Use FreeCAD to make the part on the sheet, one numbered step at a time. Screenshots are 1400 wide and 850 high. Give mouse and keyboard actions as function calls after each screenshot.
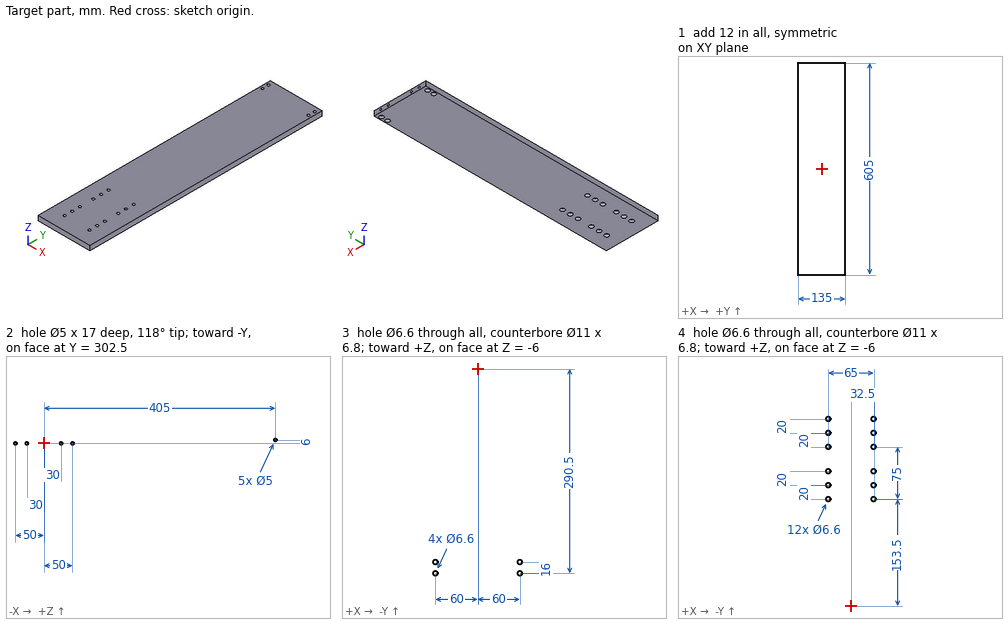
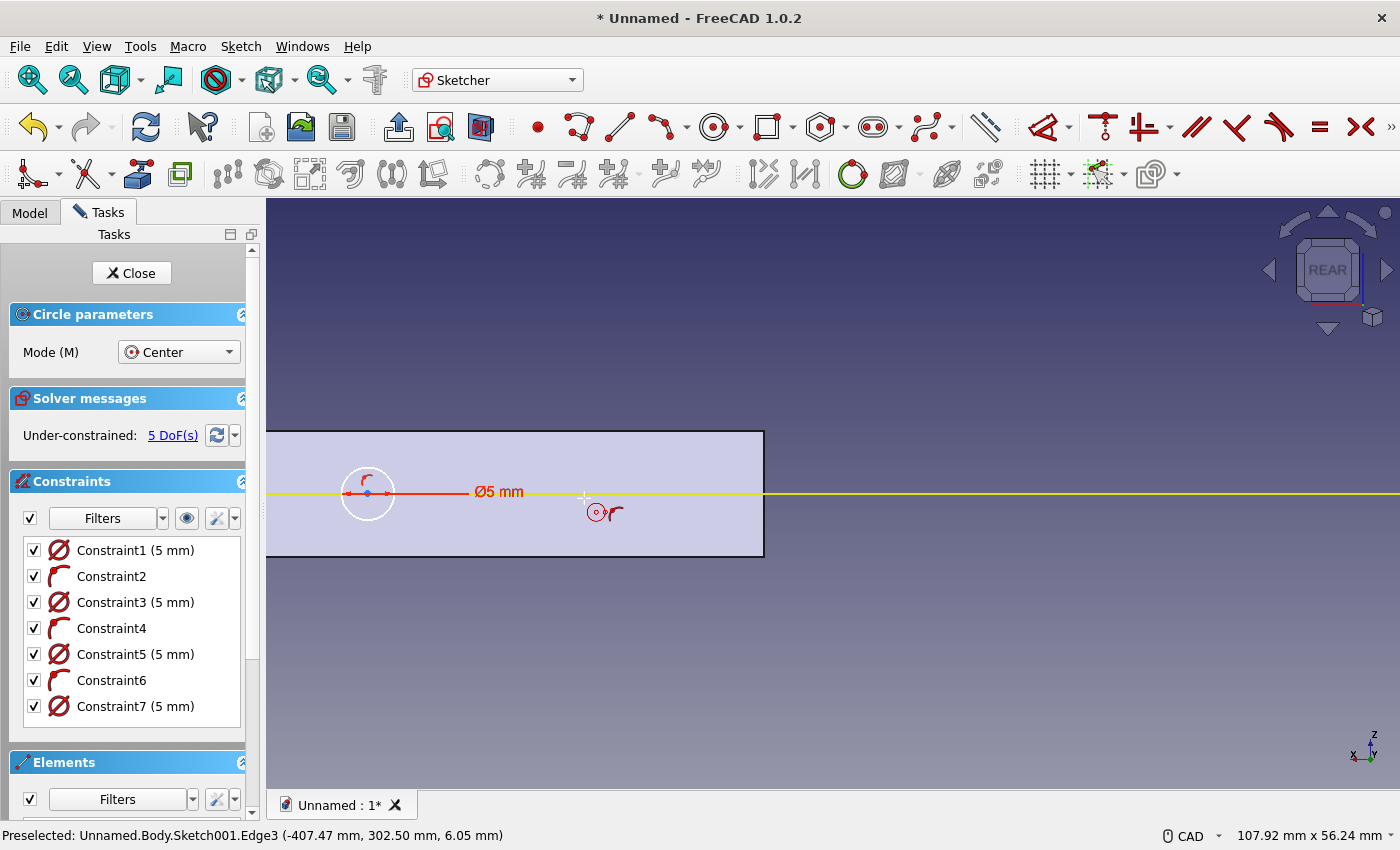
scroll(584, 498, down, 10)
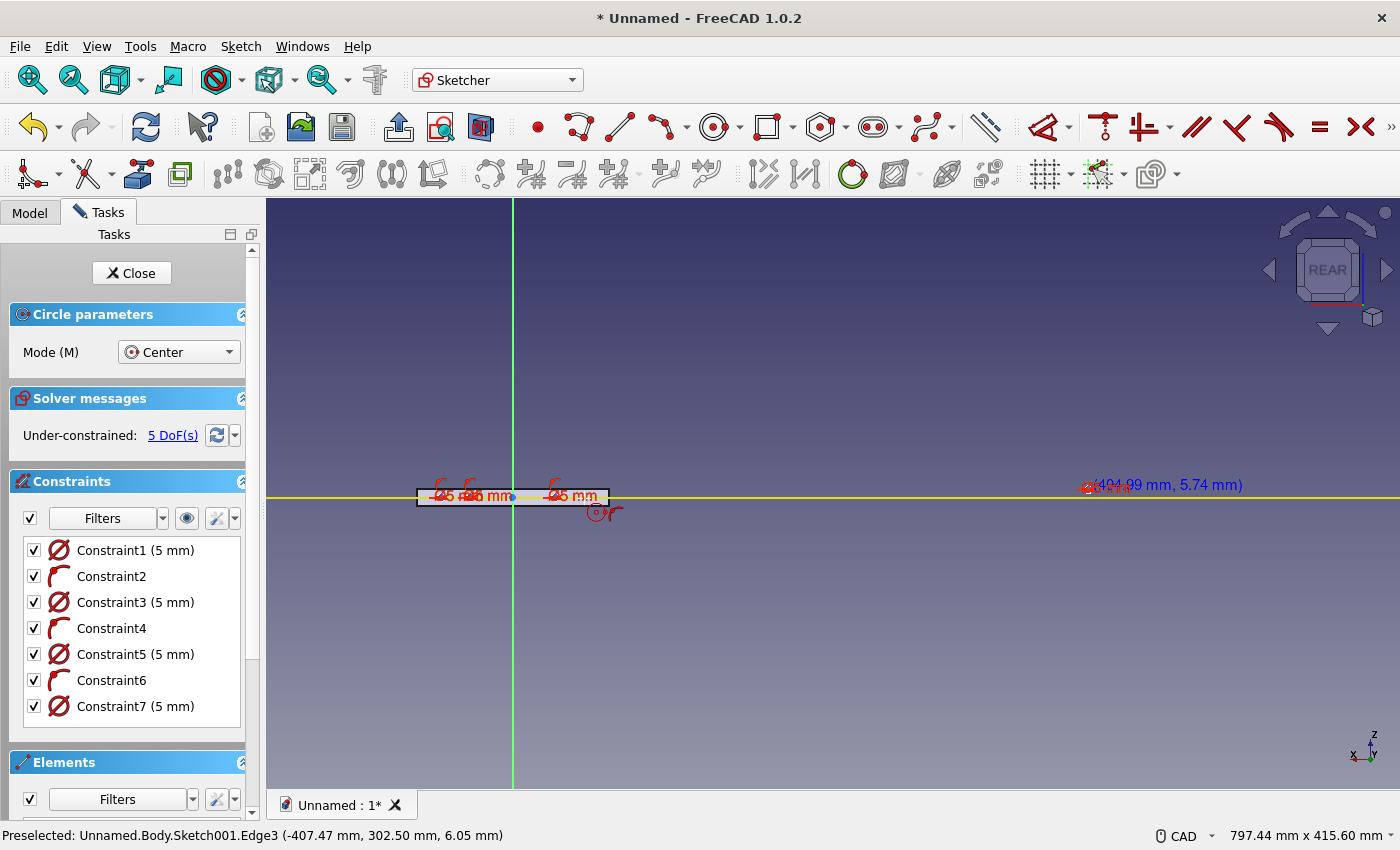
click(584, 498)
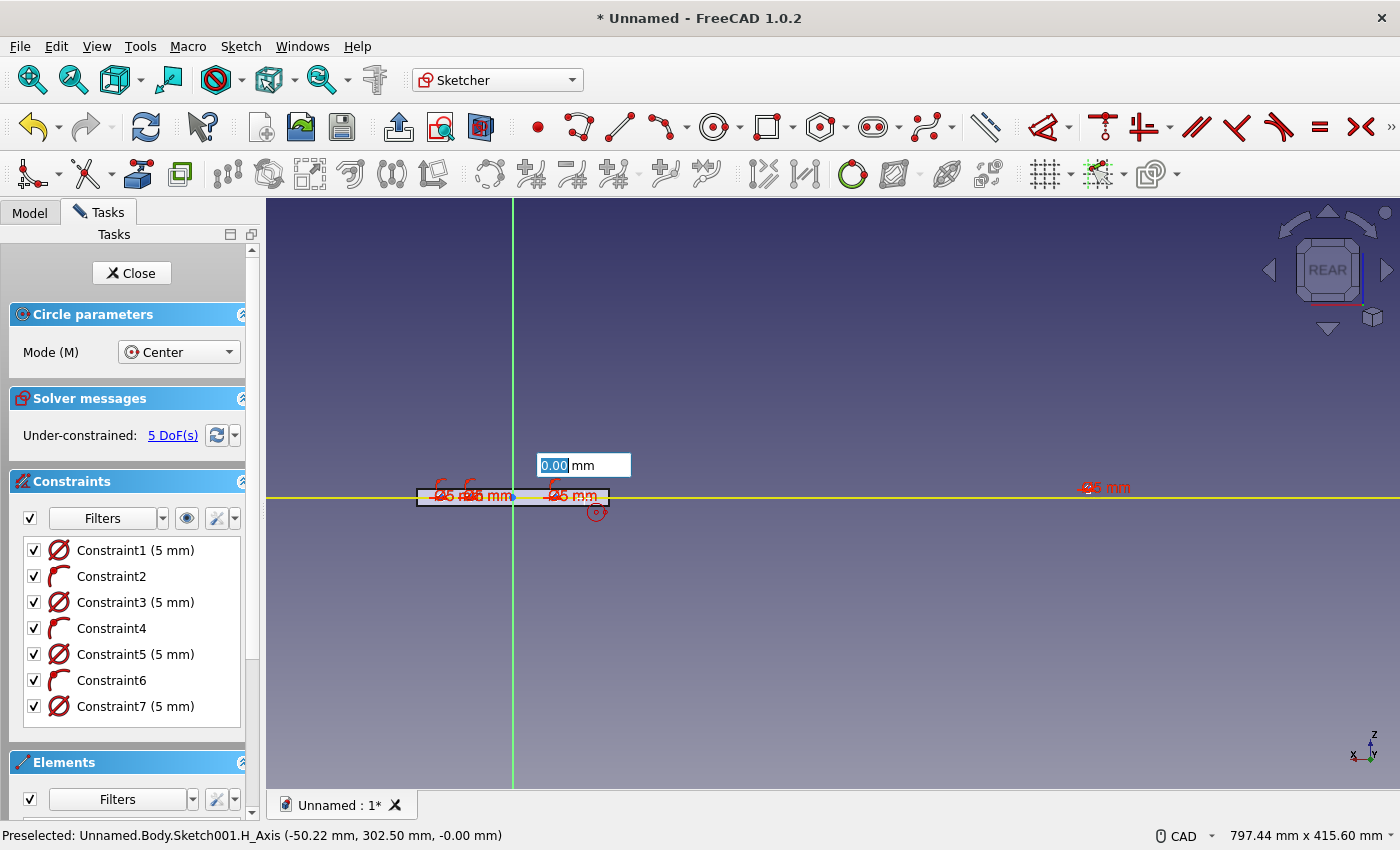
scroll(582, 501, up, 8)
move(583, 500)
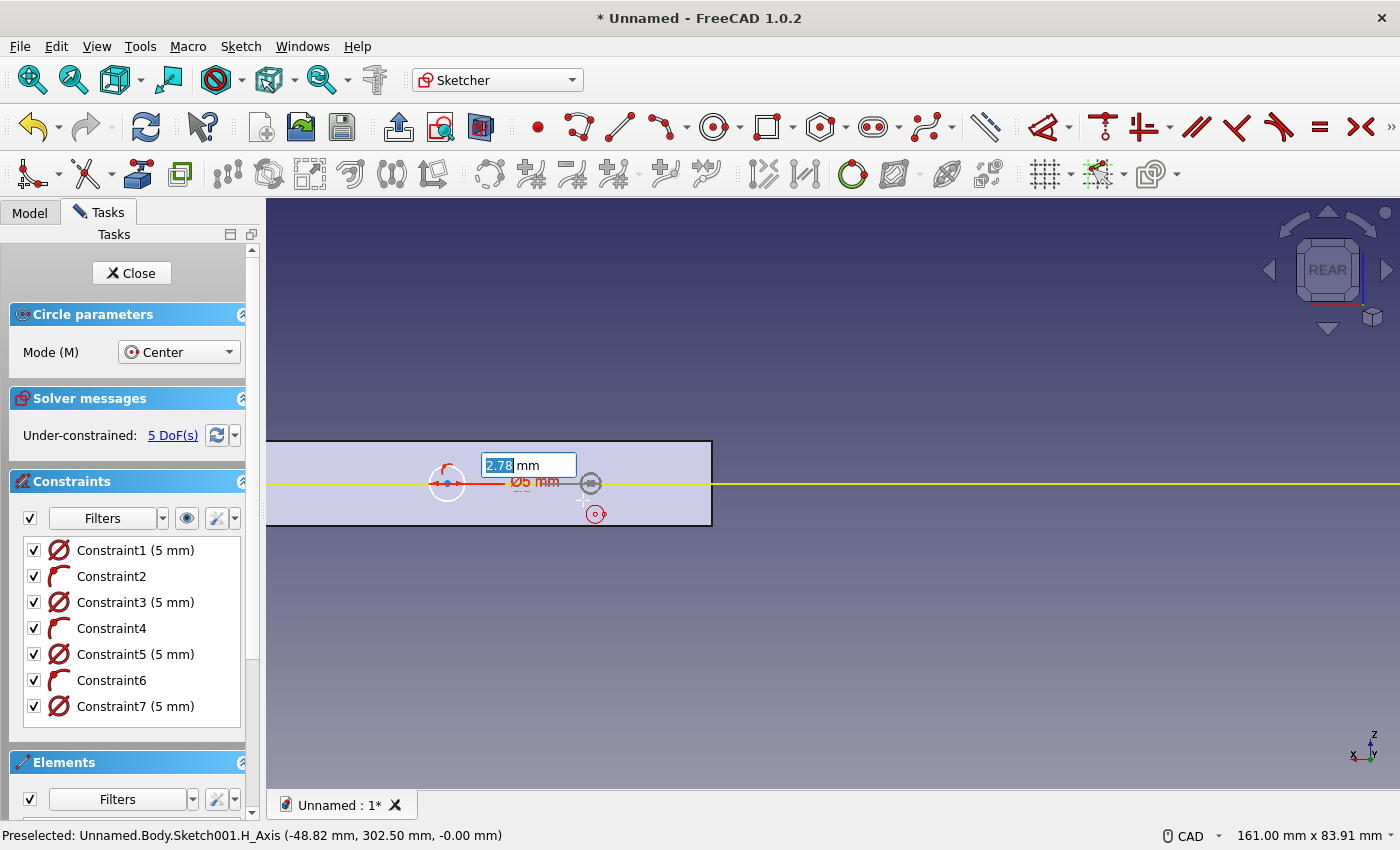
text(5)
key(Return)
key(Escape)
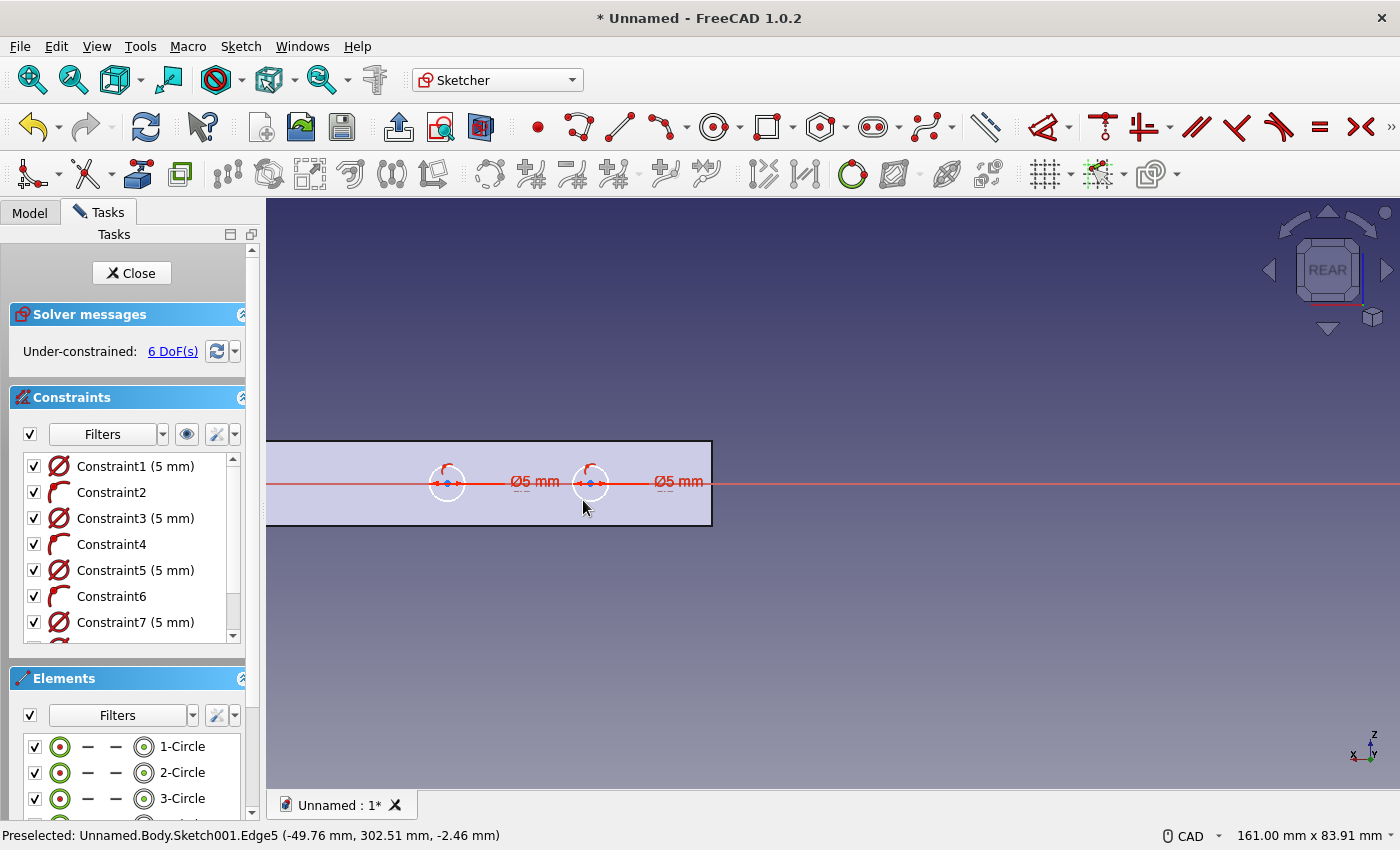
scroll(582, 501, down, 8)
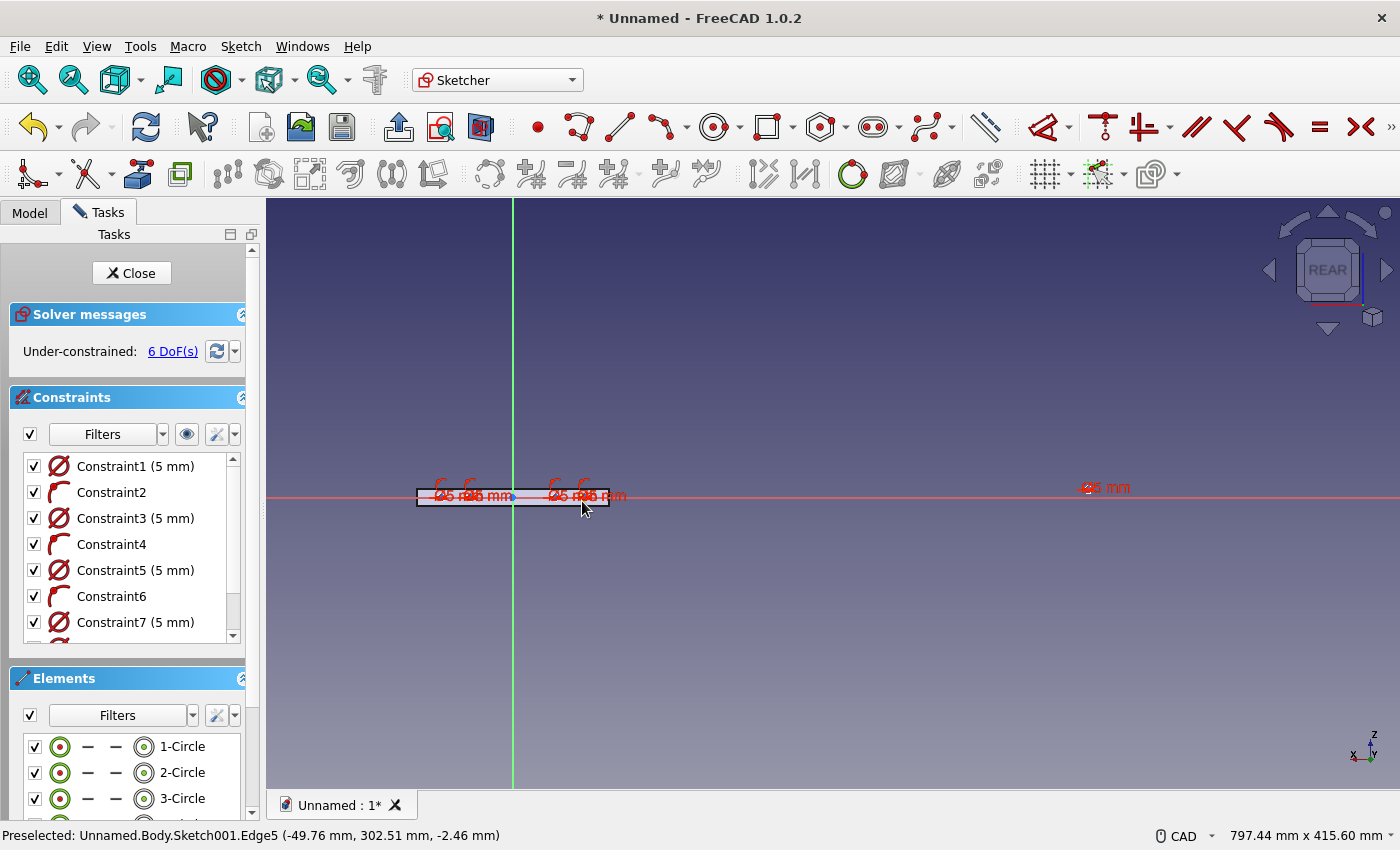
scroll(1089, 490, up, 8)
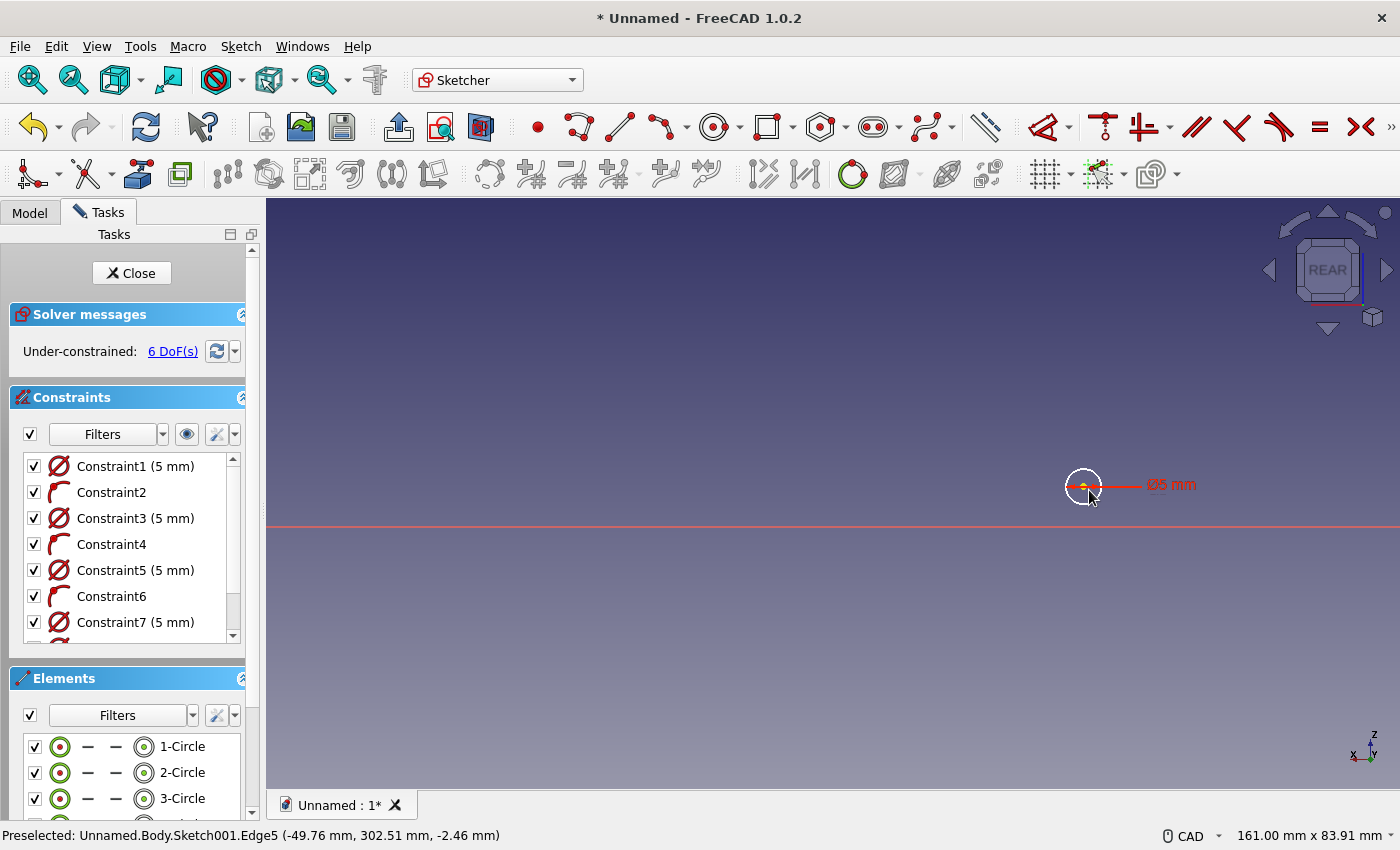
click(1084, 487)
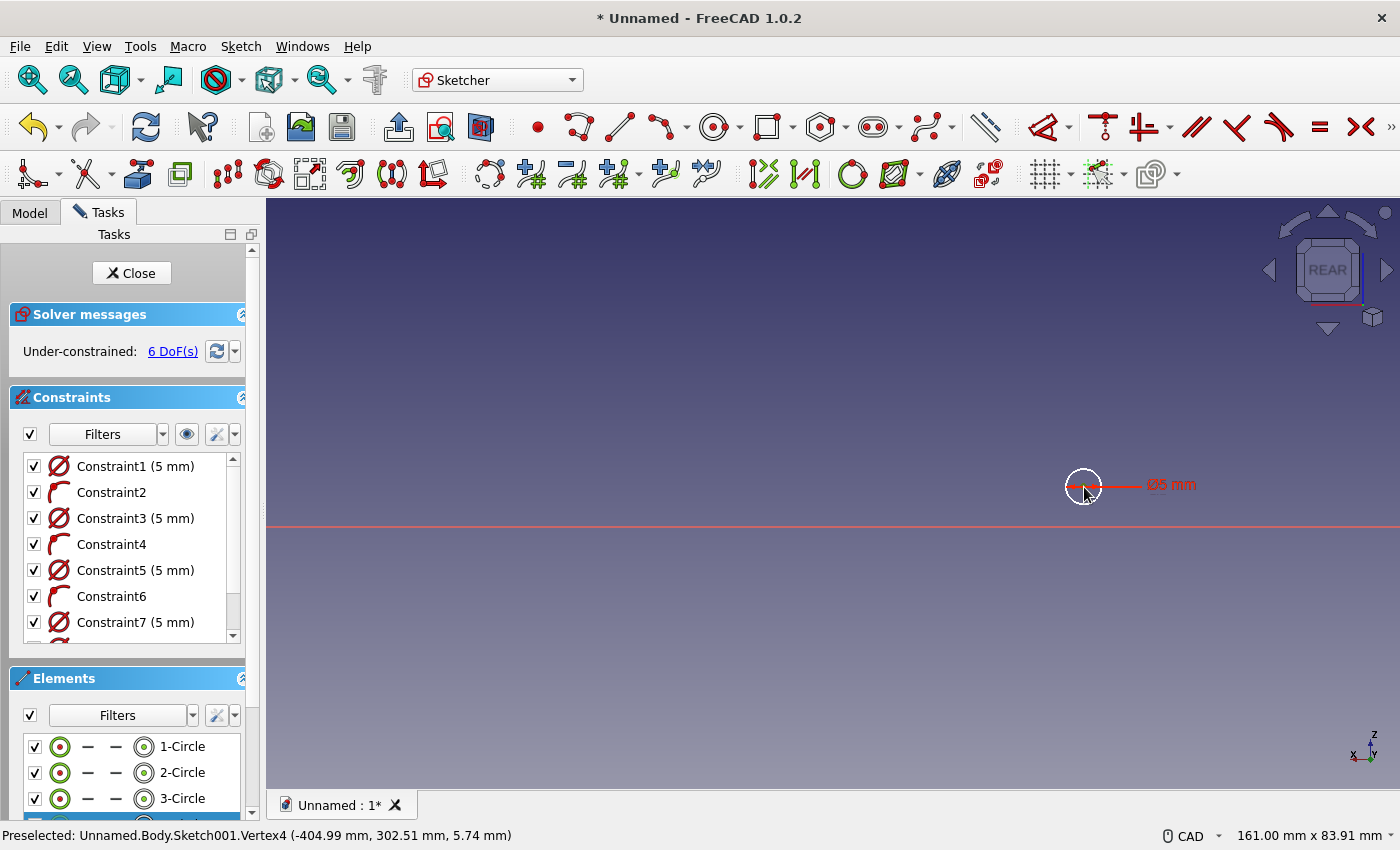
key(i)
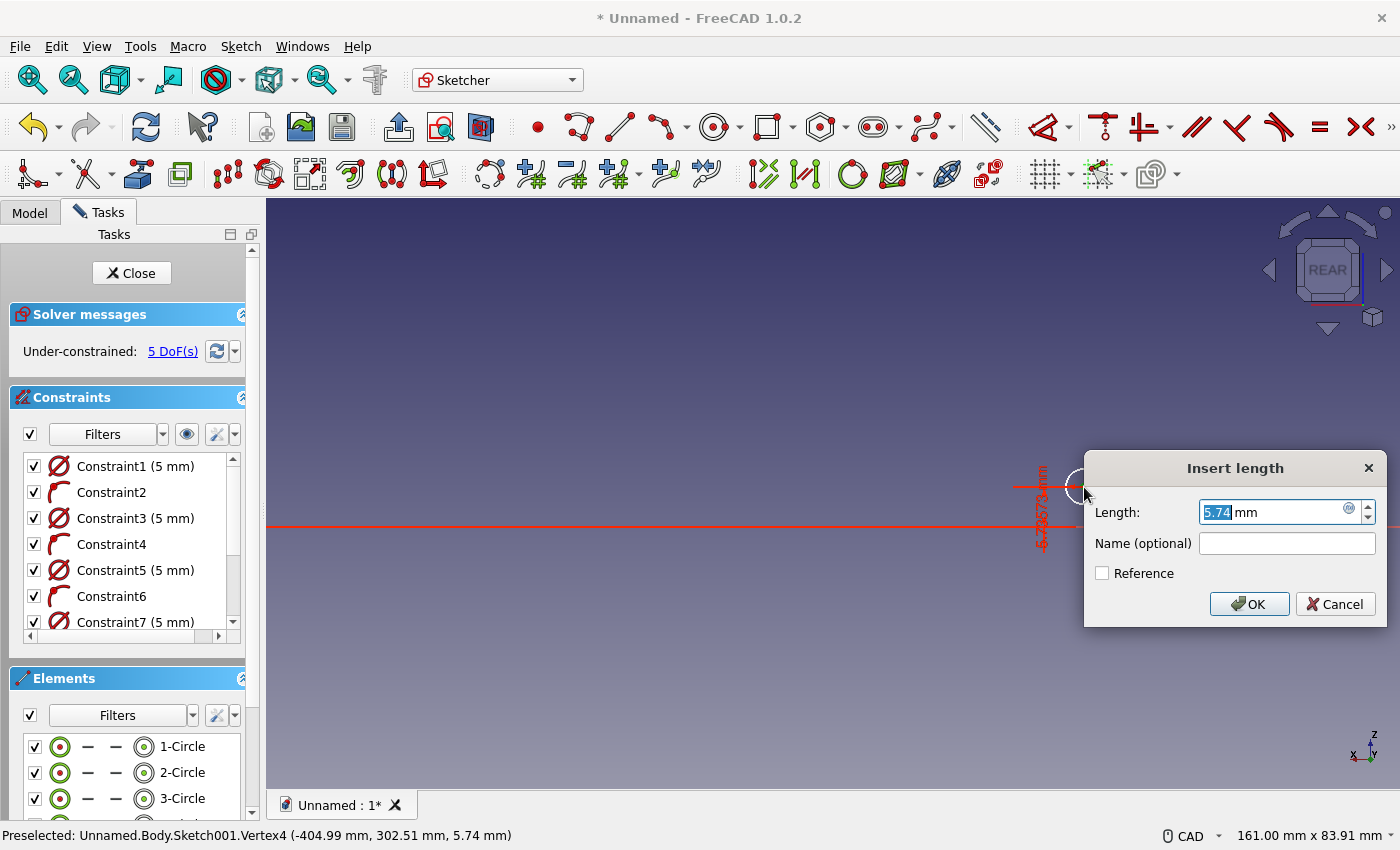
text(6)
key(Return)